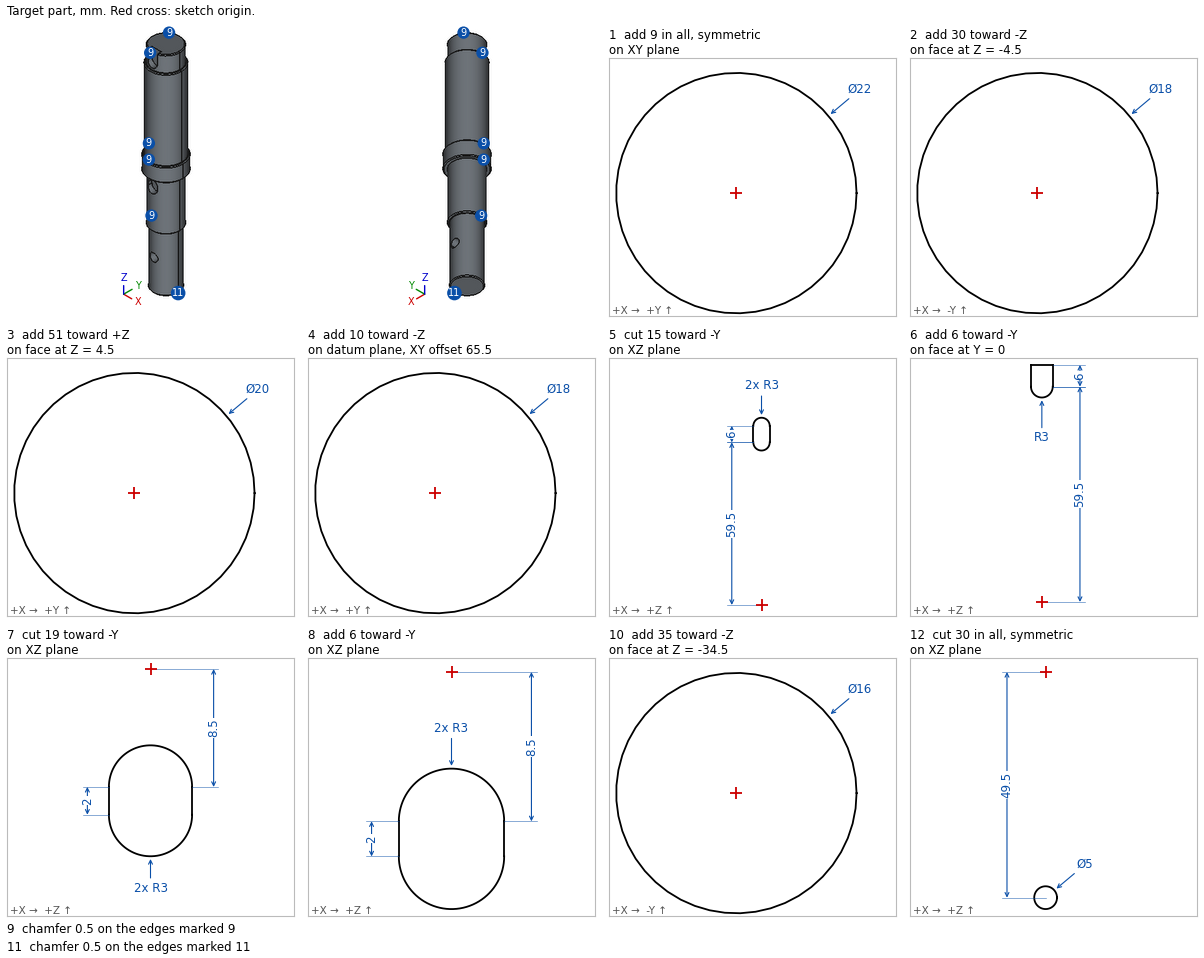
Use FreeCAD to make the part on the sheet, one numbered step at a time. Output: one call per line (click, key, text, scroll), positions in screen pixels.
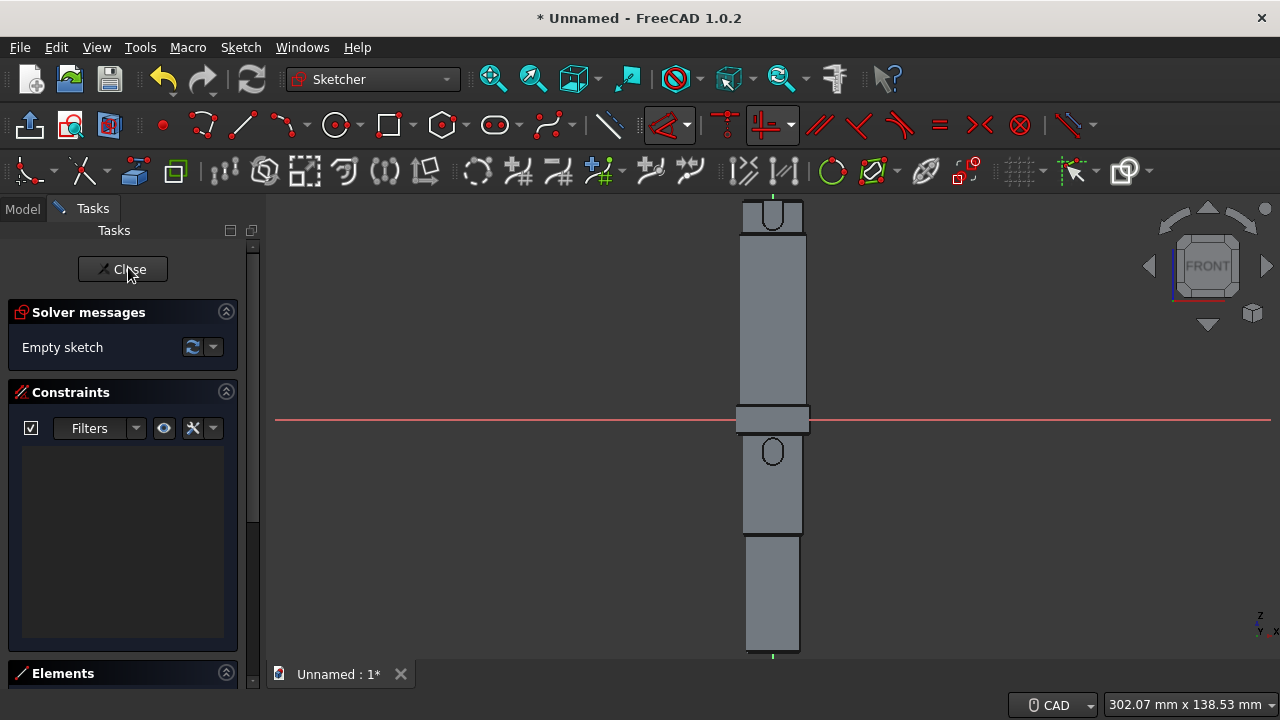
click(110, 126)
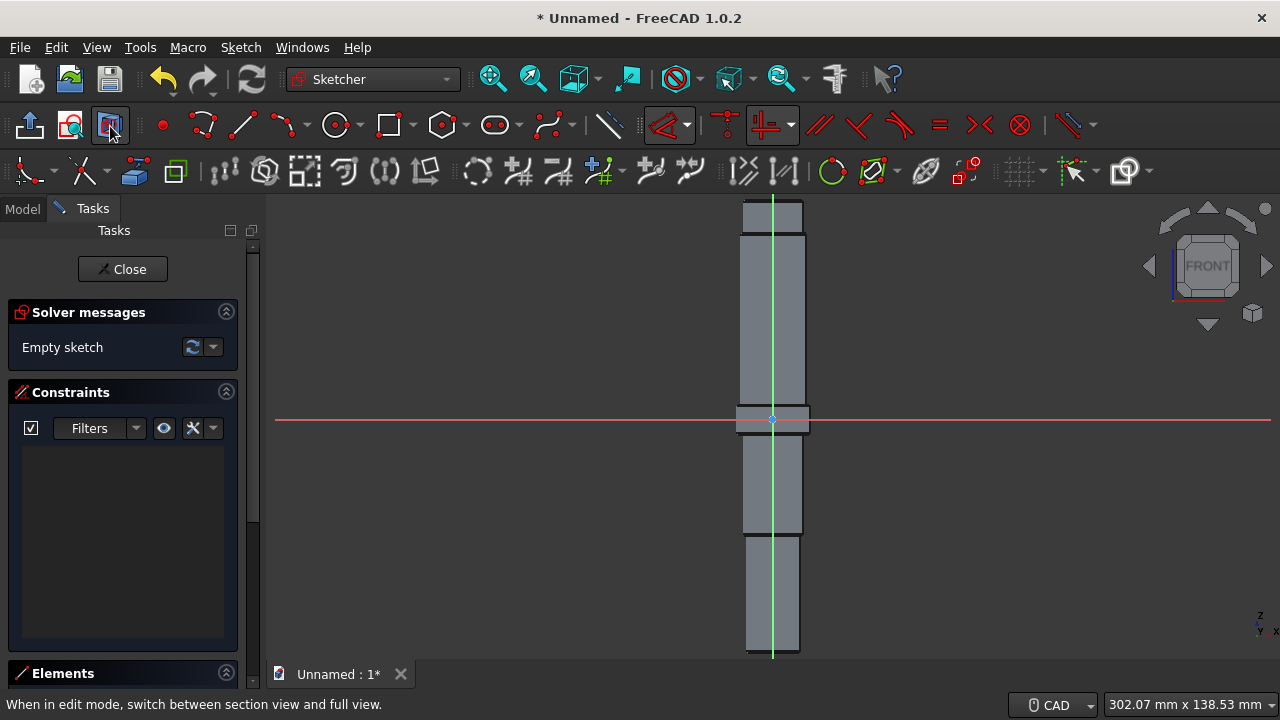
scroll(777, 596, up, 14)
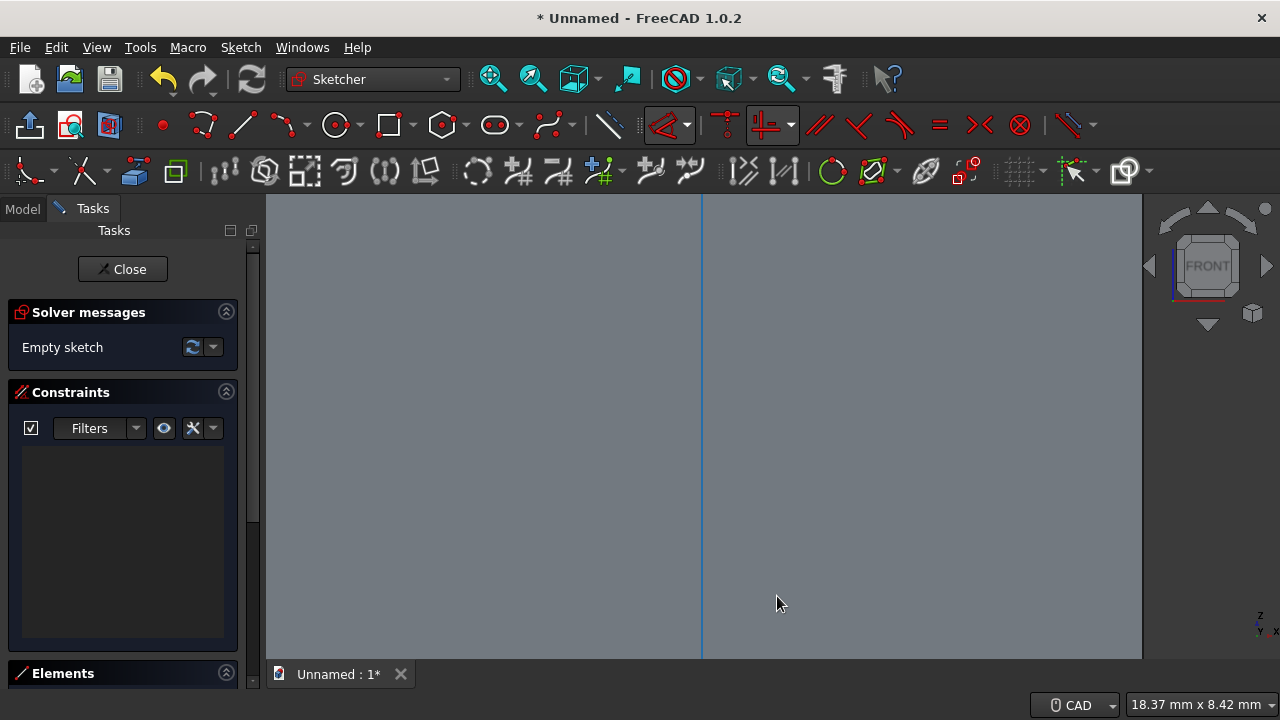
click(336, 126)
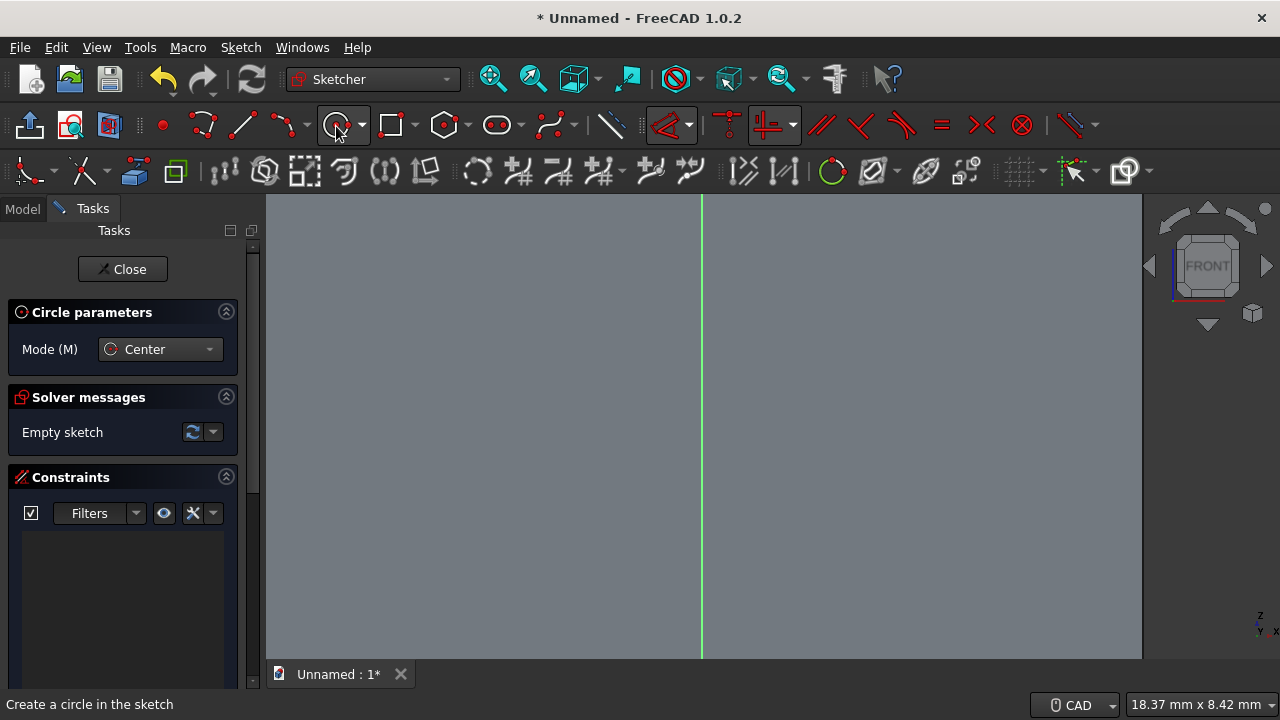
click(702, 417)
click(799, 320)
key(Escape)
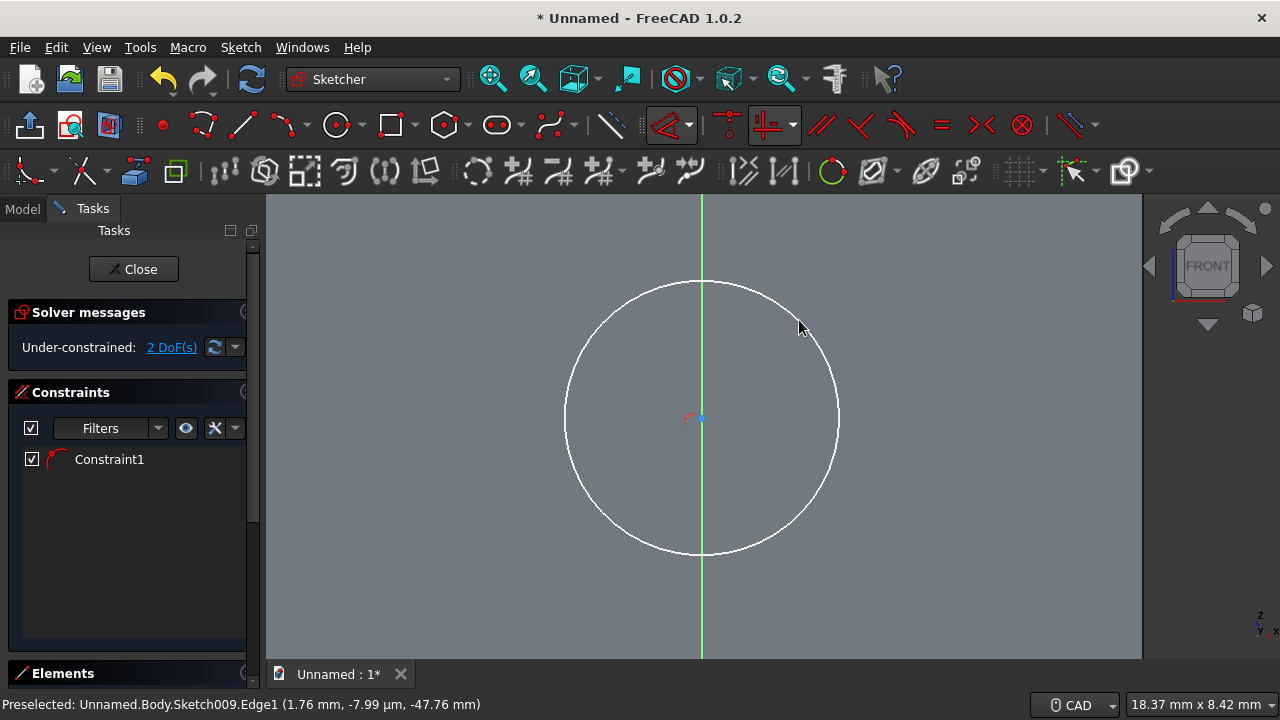
click(799, 321)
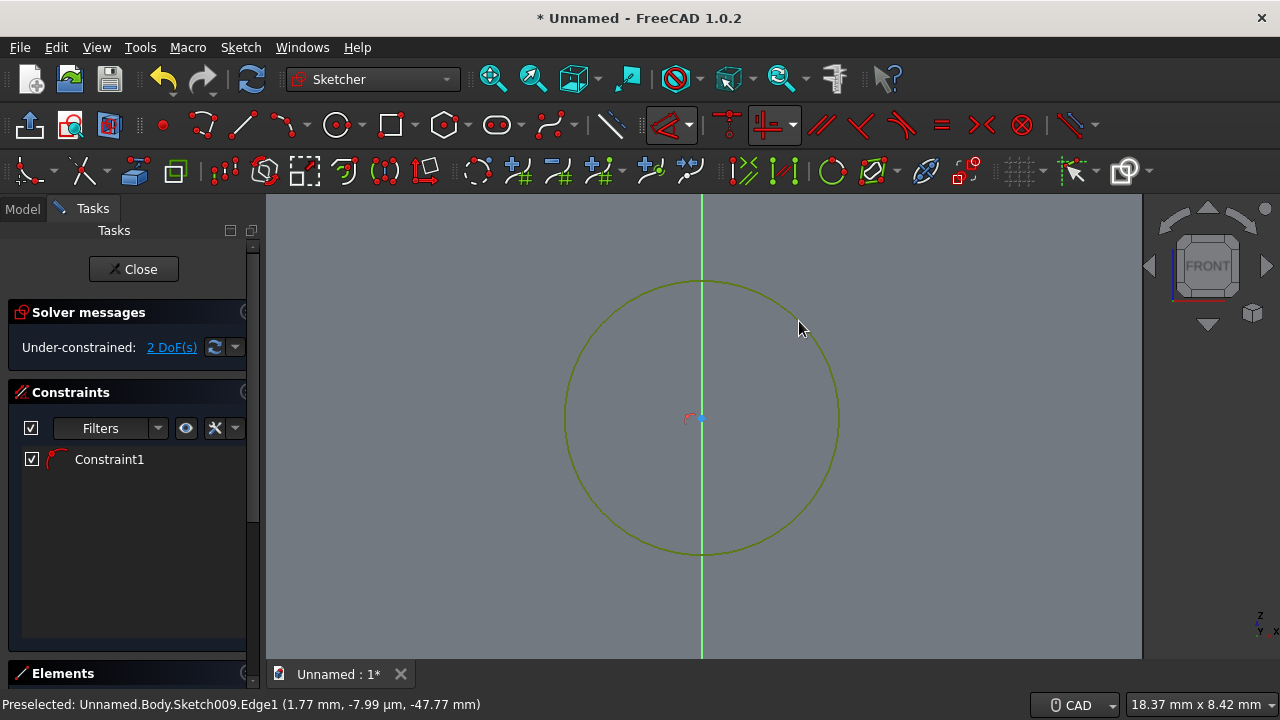
key(k)
key(o)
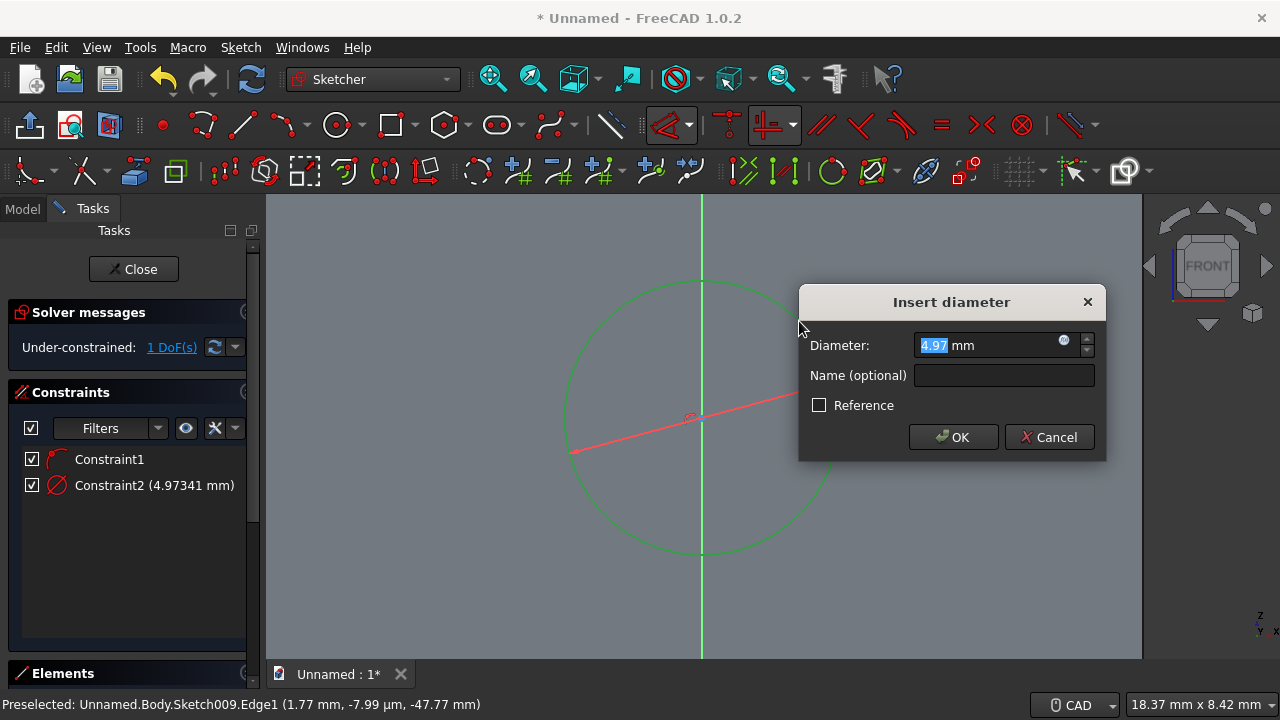
text(5)
key(Return)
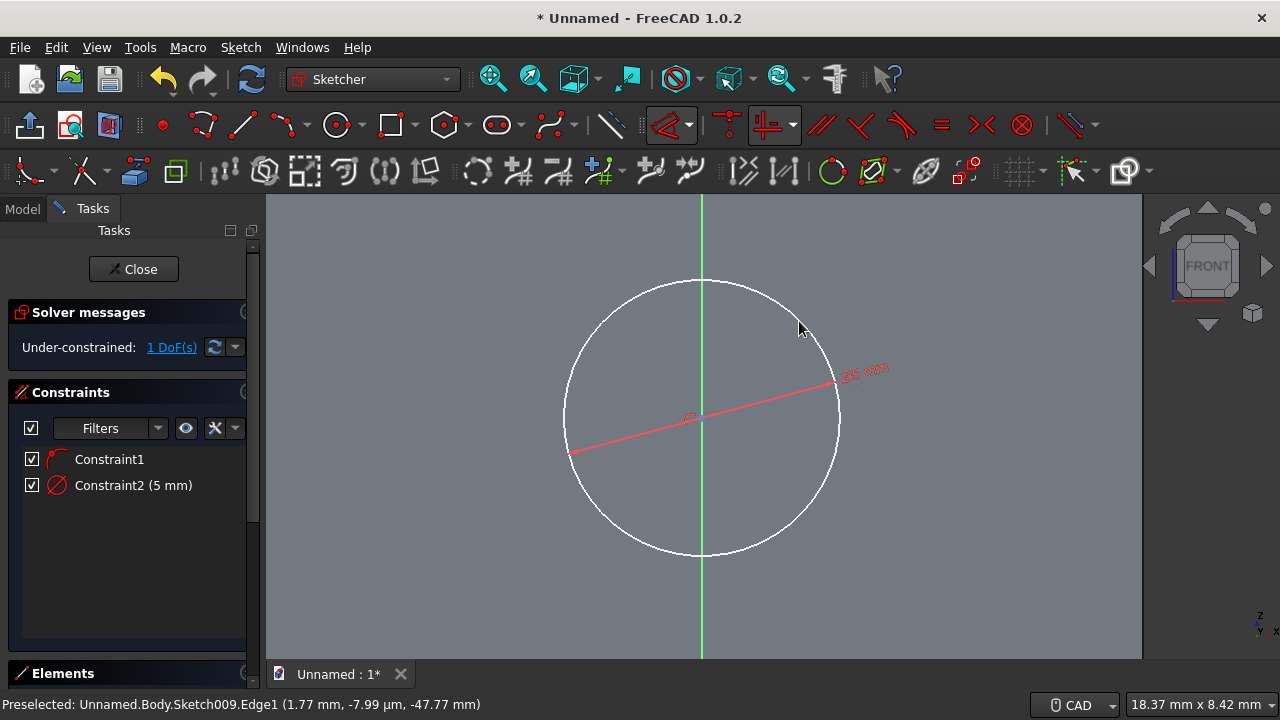
click(702, 418)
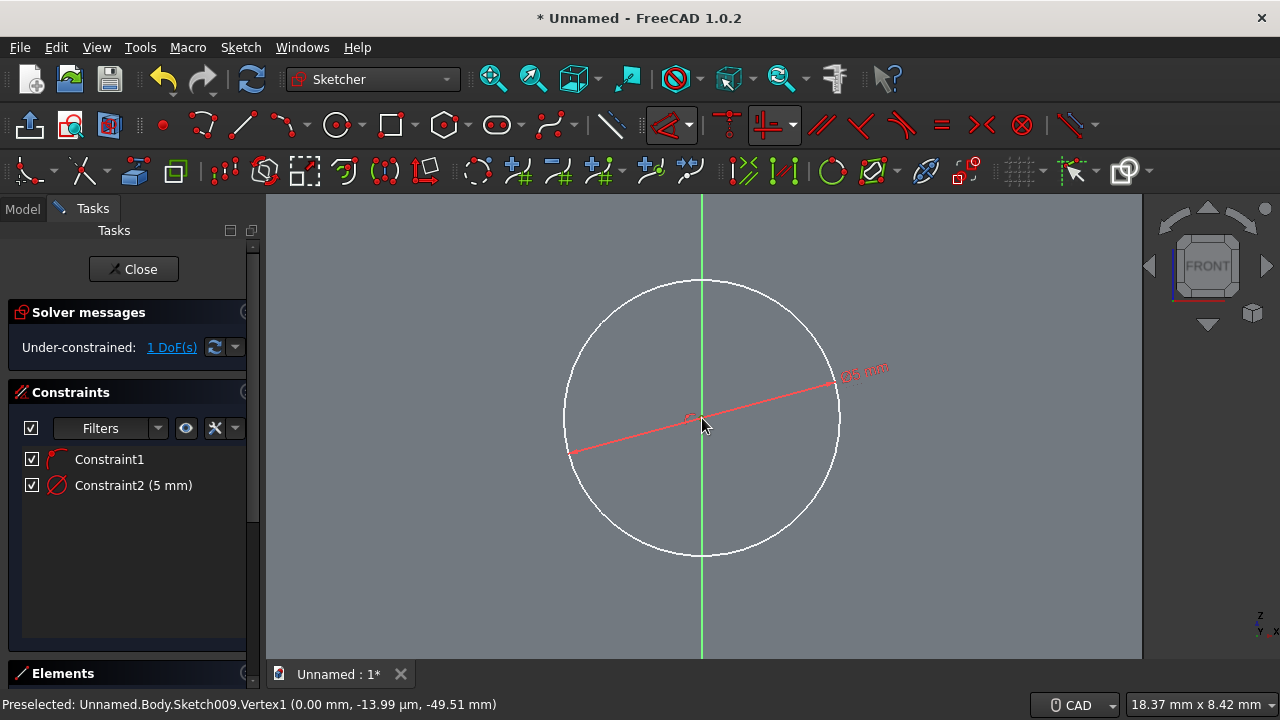
click(692, 126)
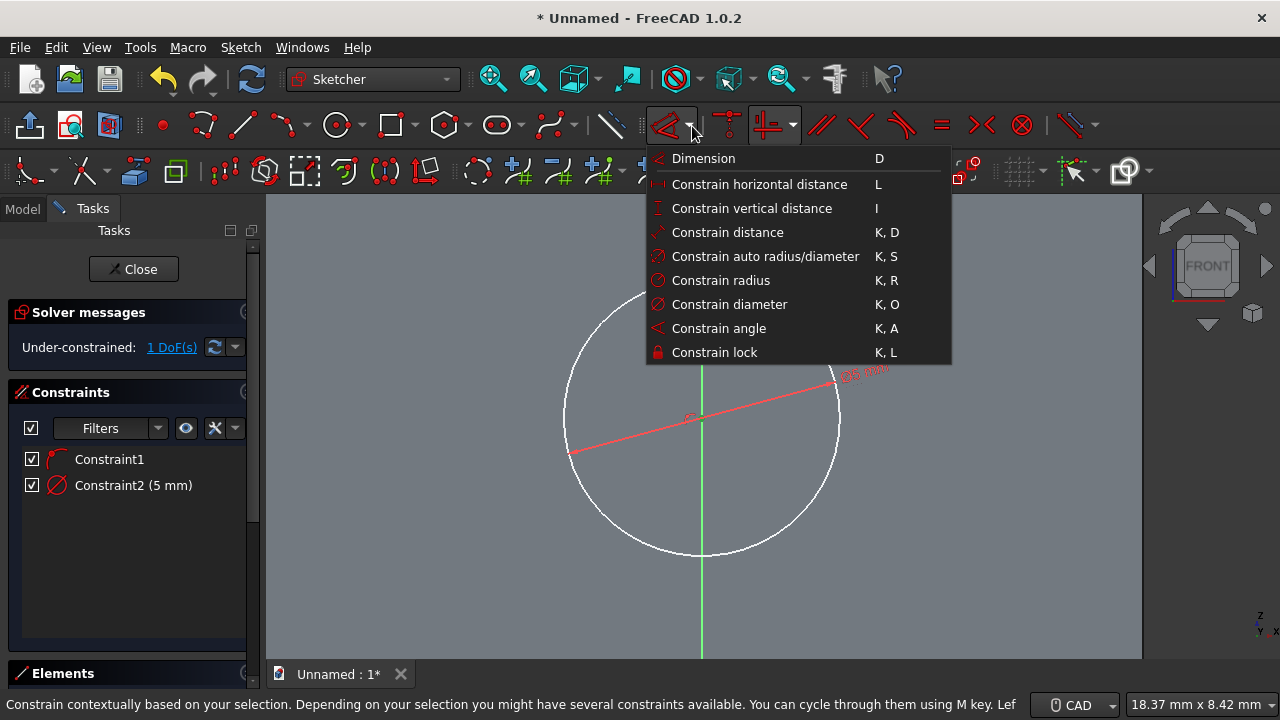
click(799, 208)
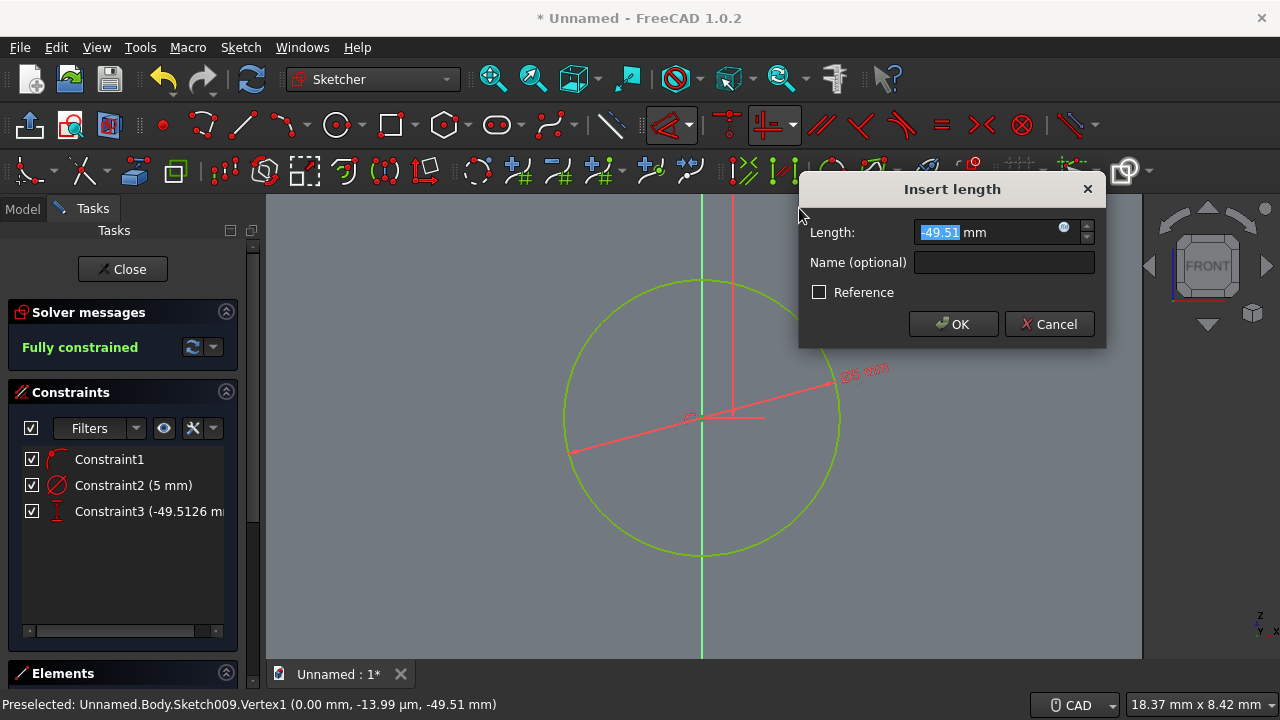
text(-49.5)
key(Return)